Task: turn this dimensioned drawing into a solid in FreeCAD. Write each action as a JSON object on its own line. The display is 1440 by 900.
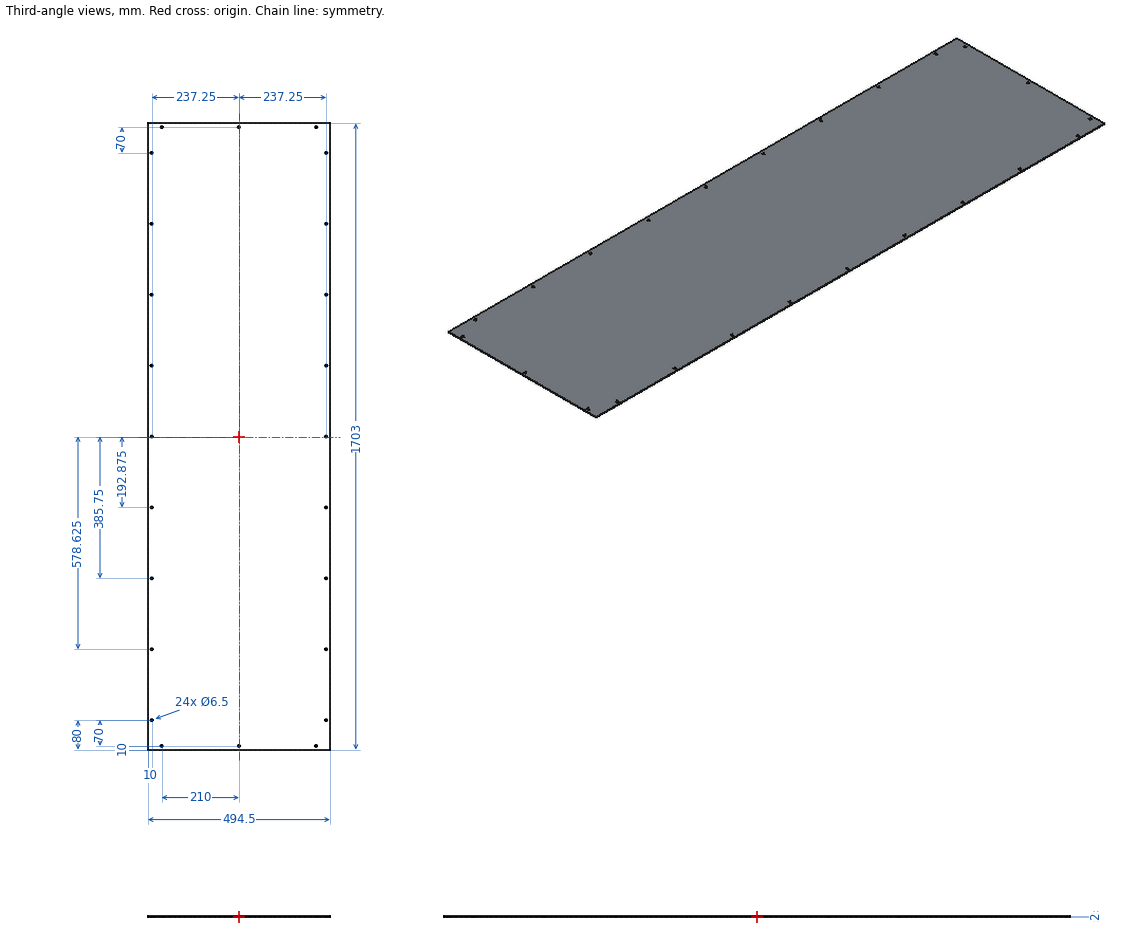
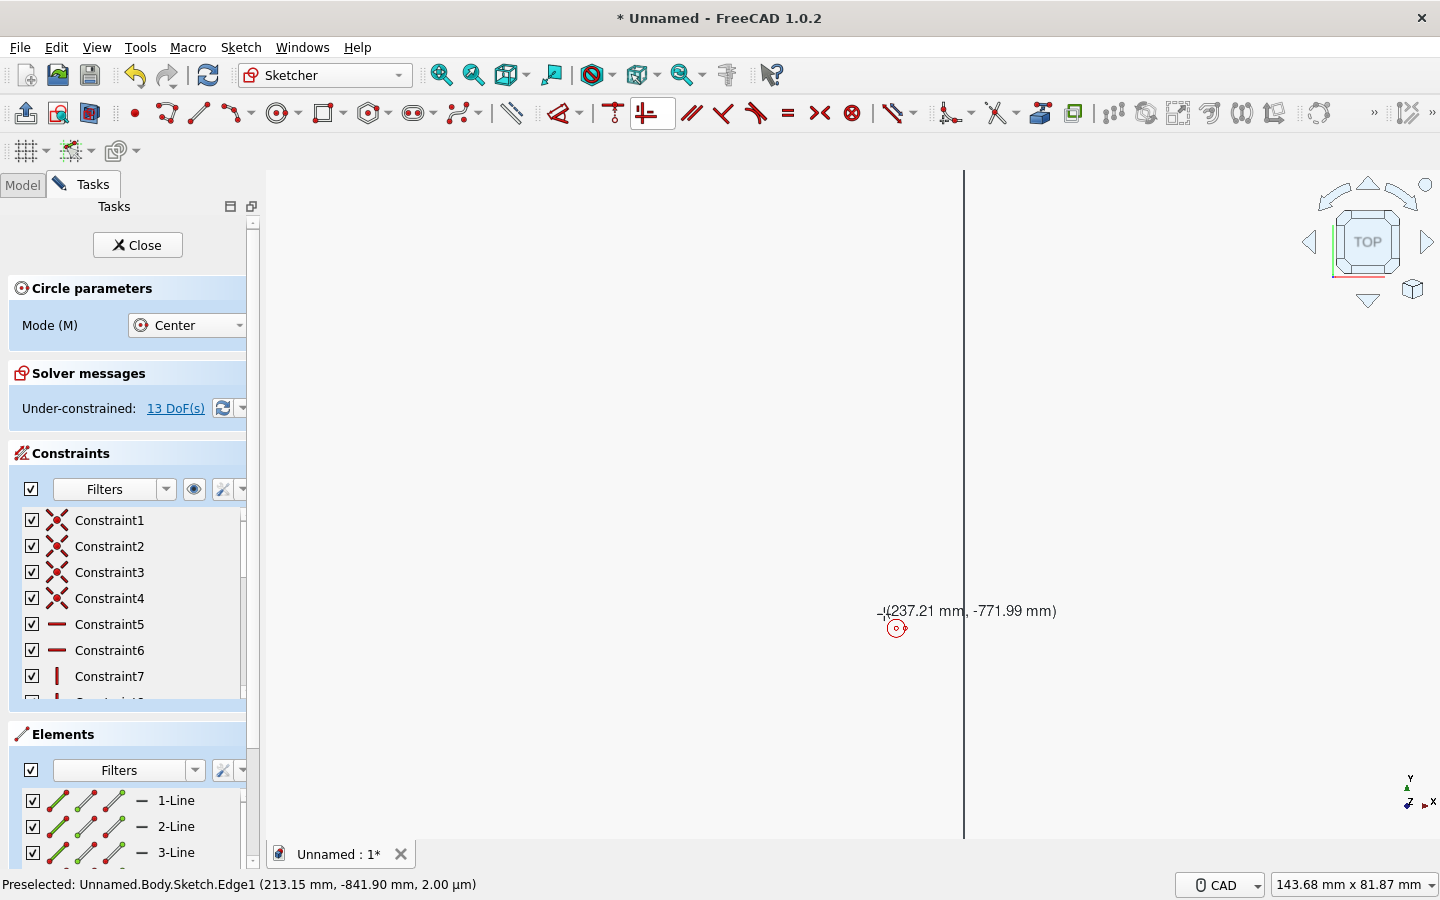
{"action": "scroll", "coordinate": [848, 718], "scroll_direction": "down", "scroll_amount": 17}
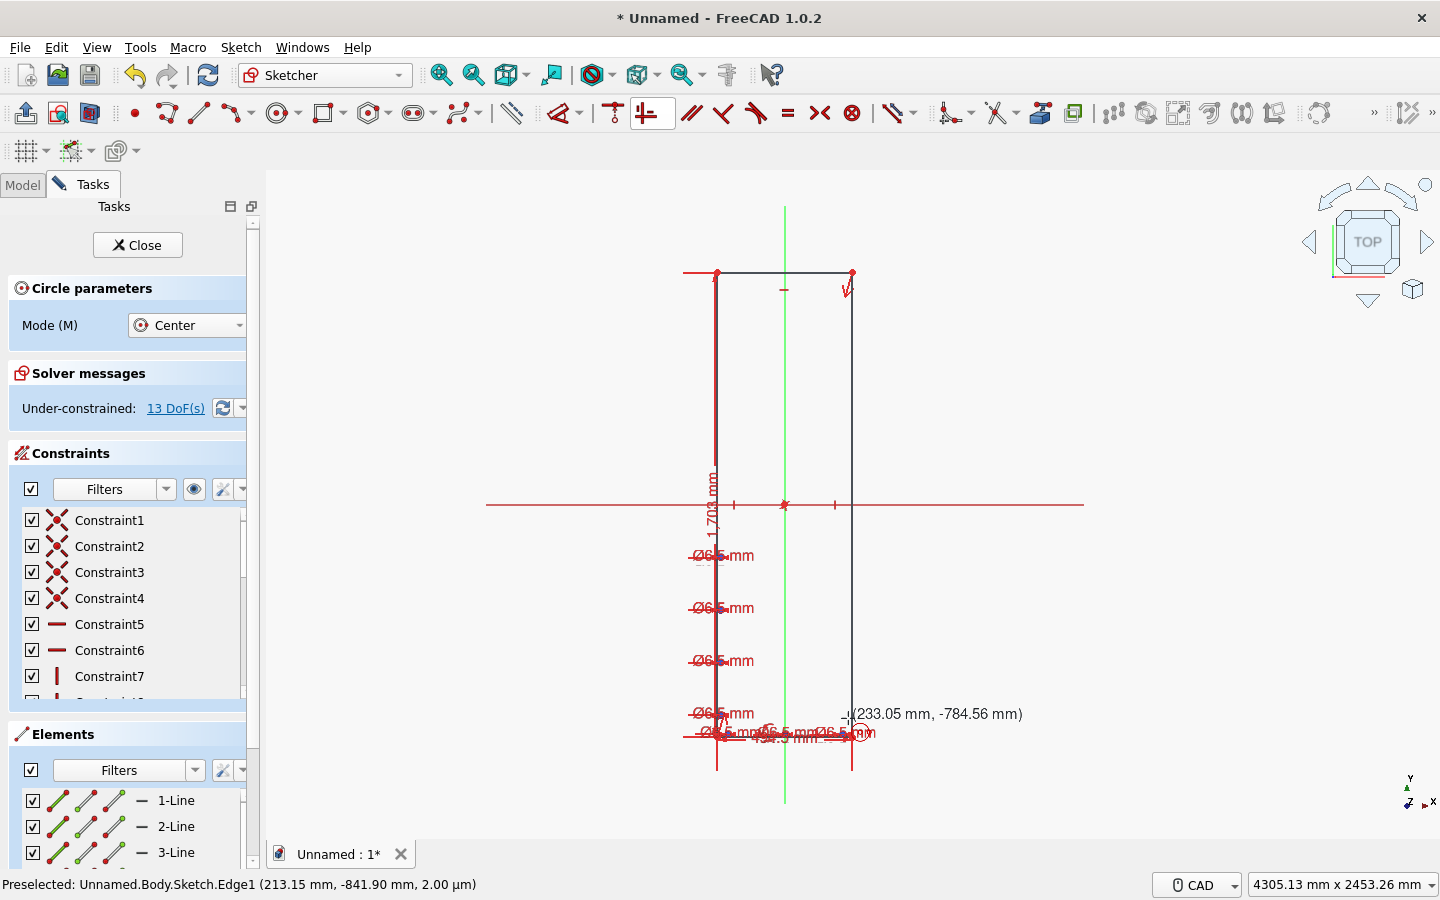
{"action": "scroll", "coordinate": [850, 715], "scroll_direction": "up", "scroll_amount": 9}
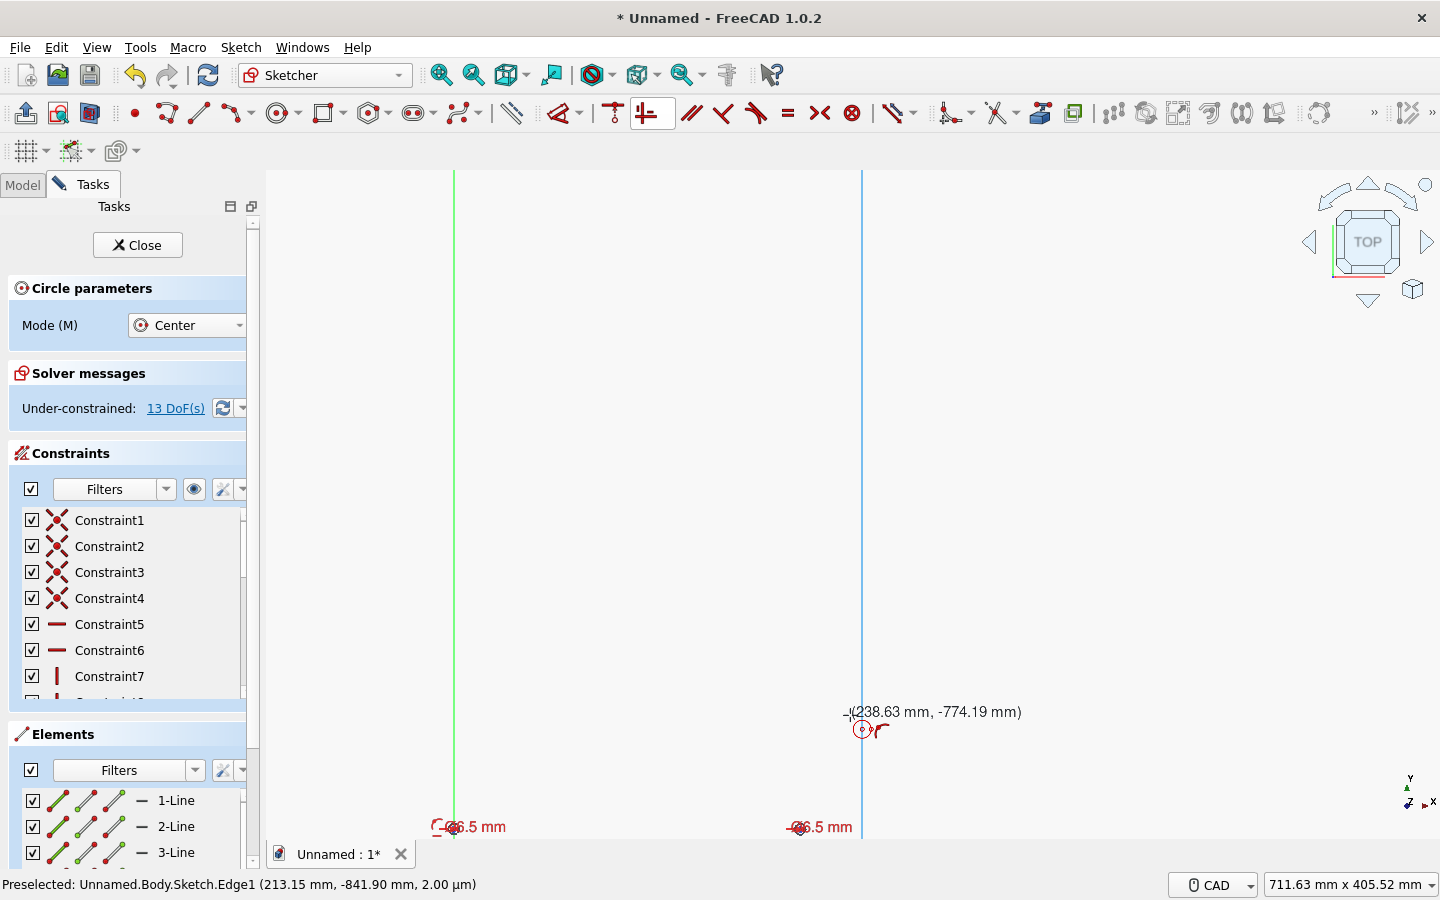
{"action": "left_click", "coordinate": [845, 712]}
{"action": "mouse_move", "coordinate": [841, 709]}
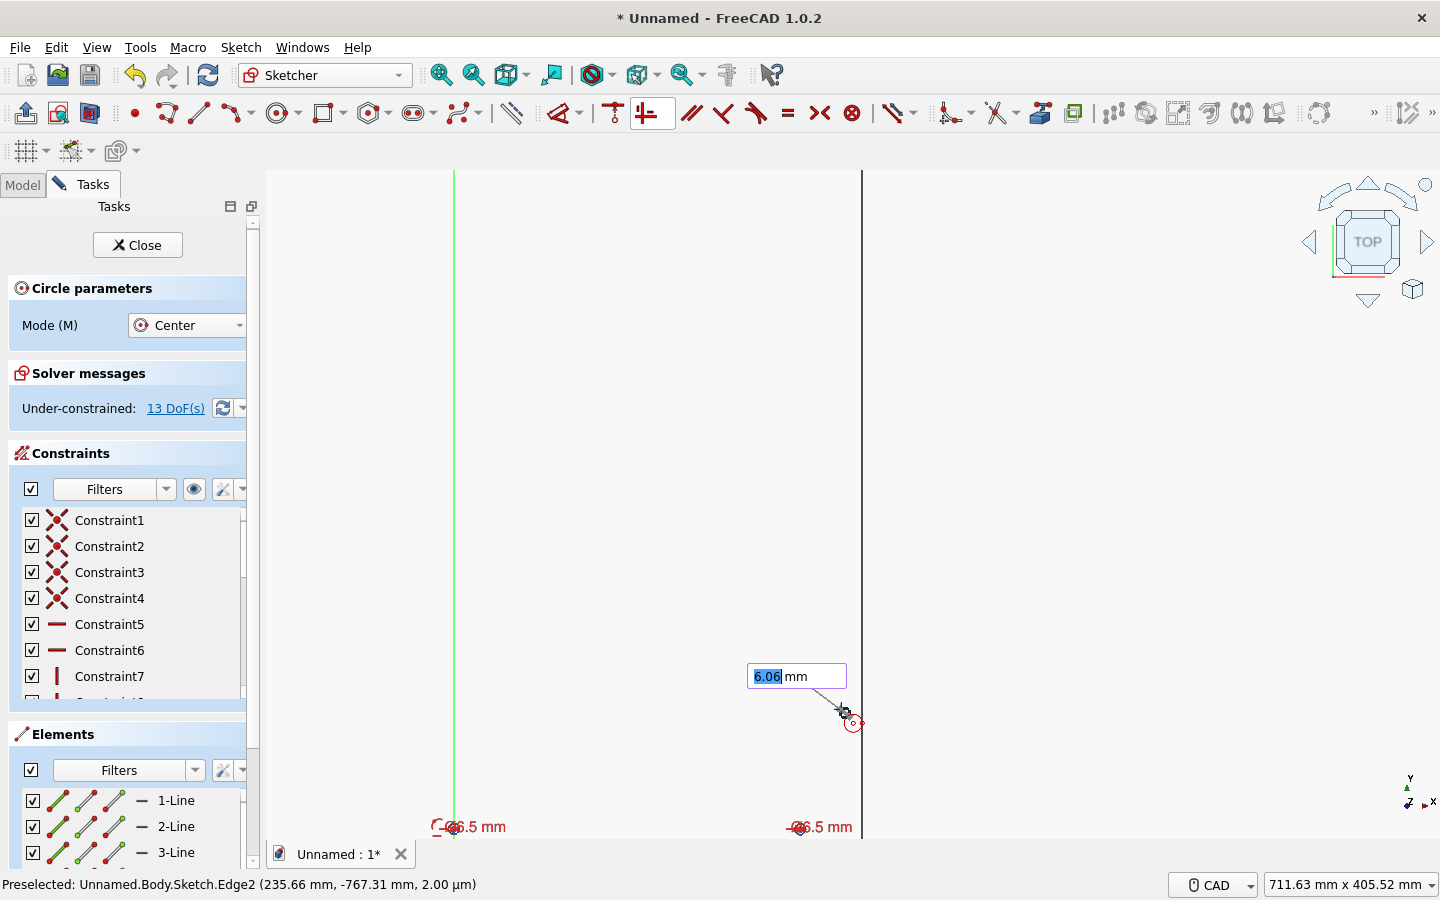
{"action": "type", "text": "6.5"}
{"action": "key", "text": "Return"}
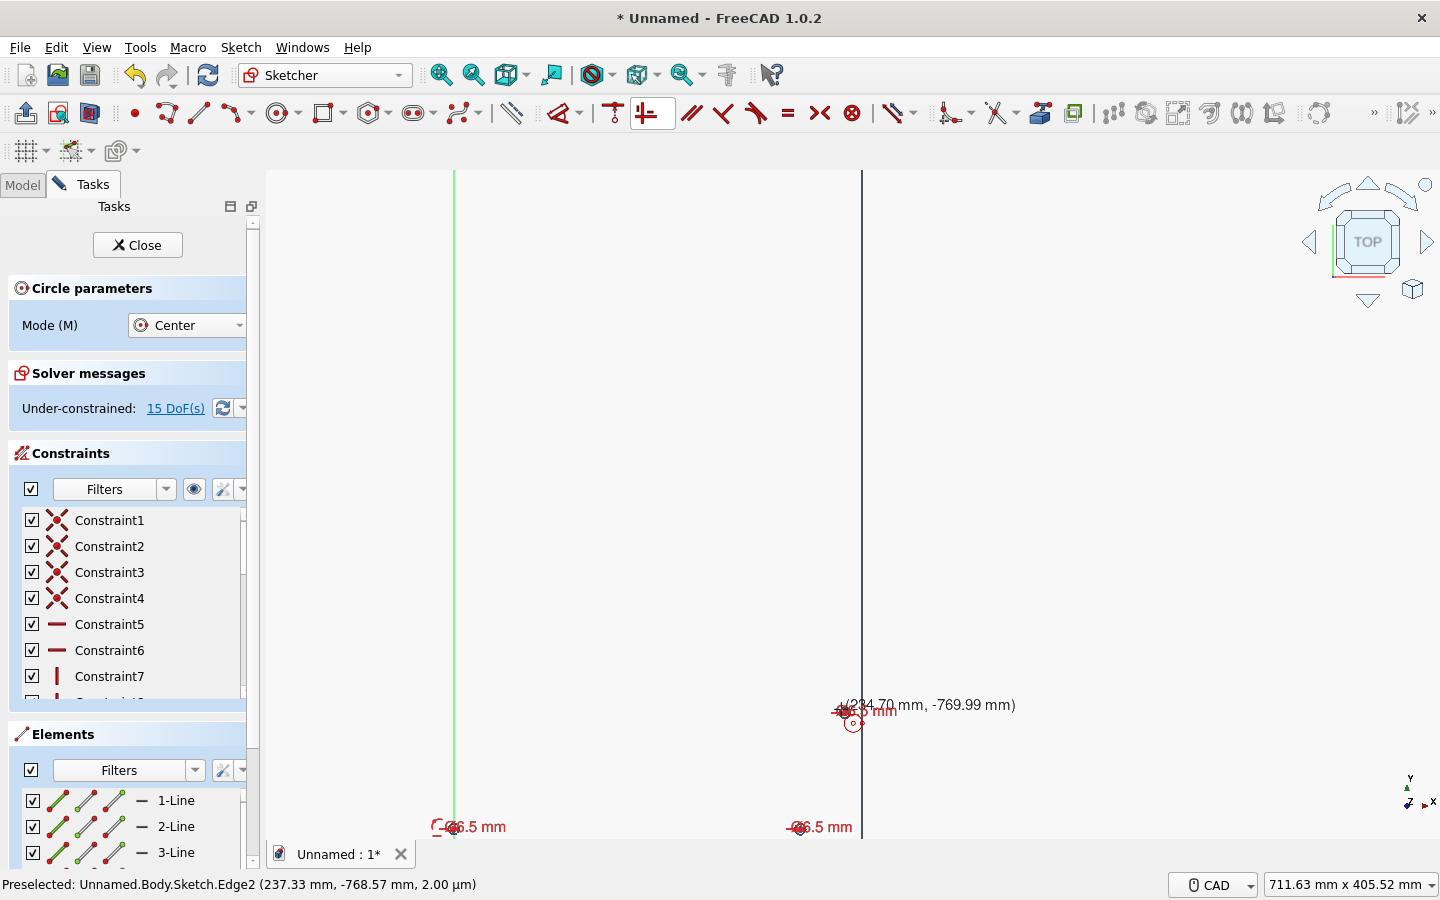
{"action": "scroll", "coordinate": [845, 394], "scroll_direction": "up", "scroll_amount": 8}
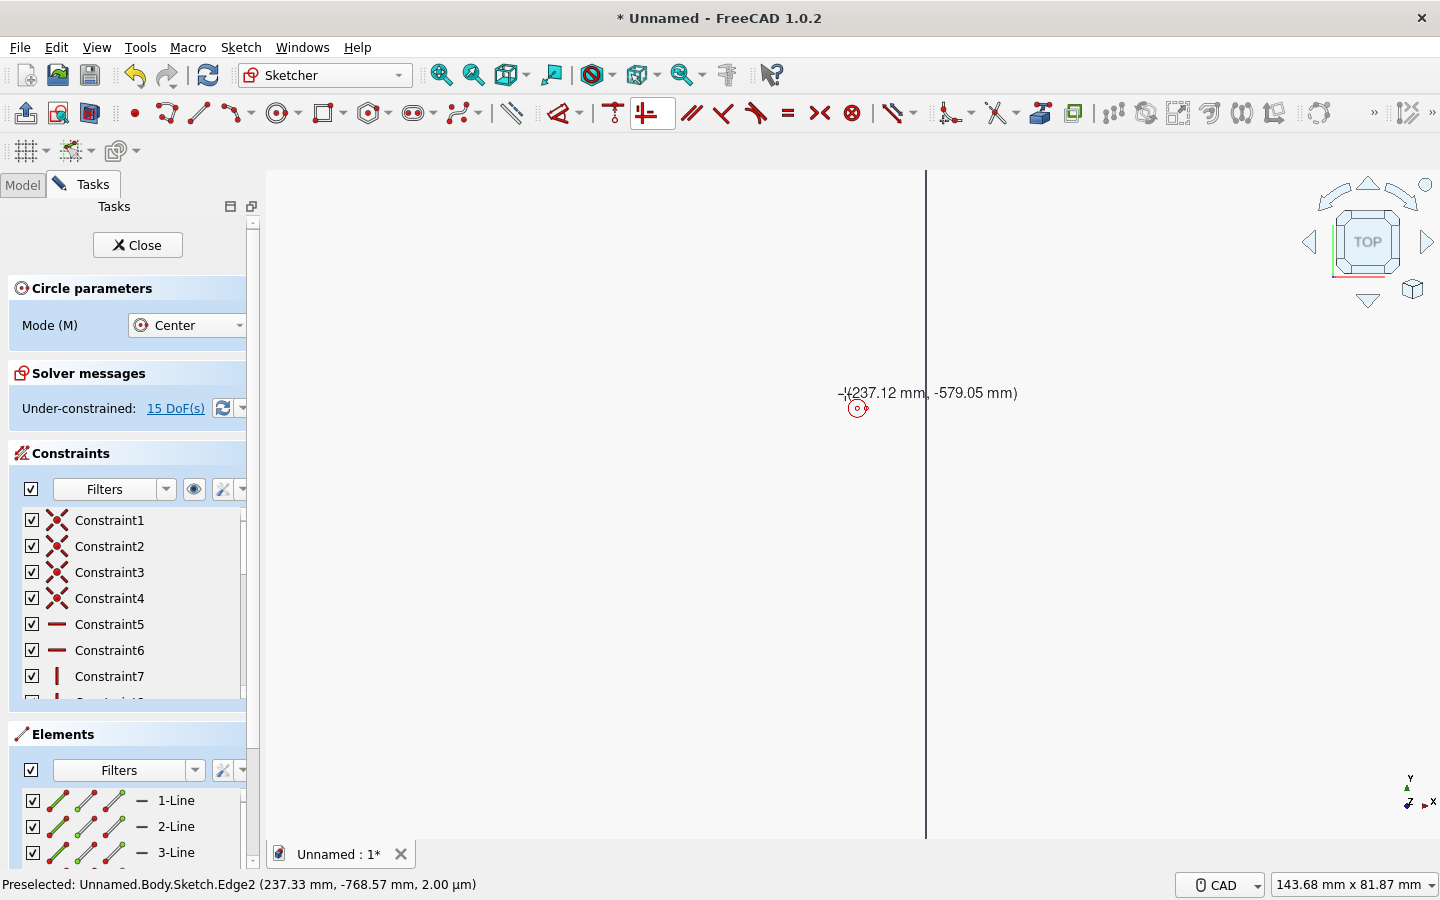
{"action": "scroll", "coordinate": [849, 672], "scroll_direction": "down", "scroll_amount": 17}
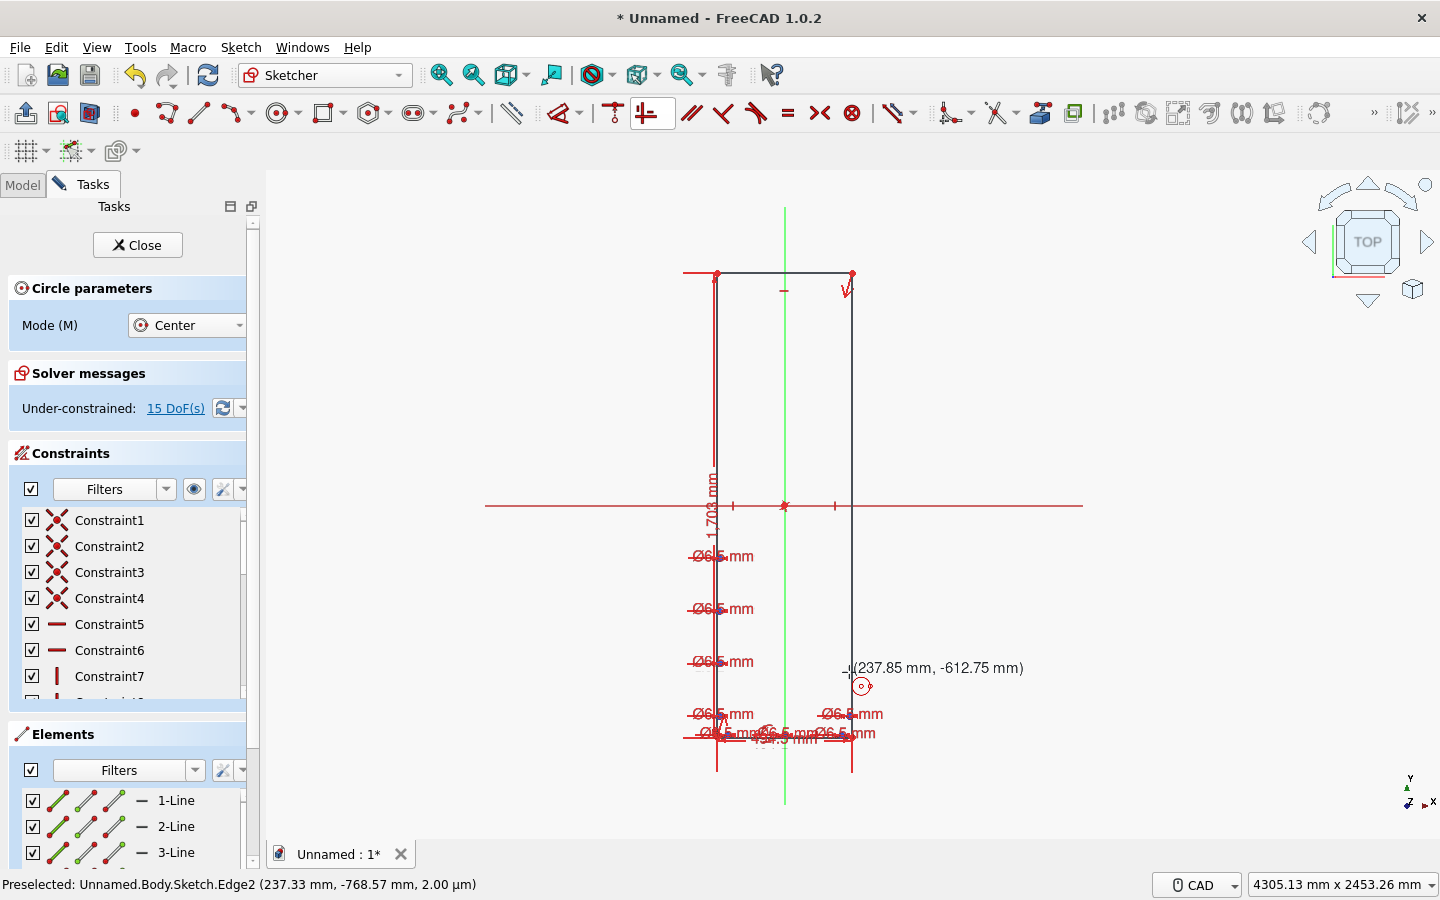
{"action": "scroll", "coordinate": [849, 663], "scroll_direction": "up", "scroll_amount": 9}